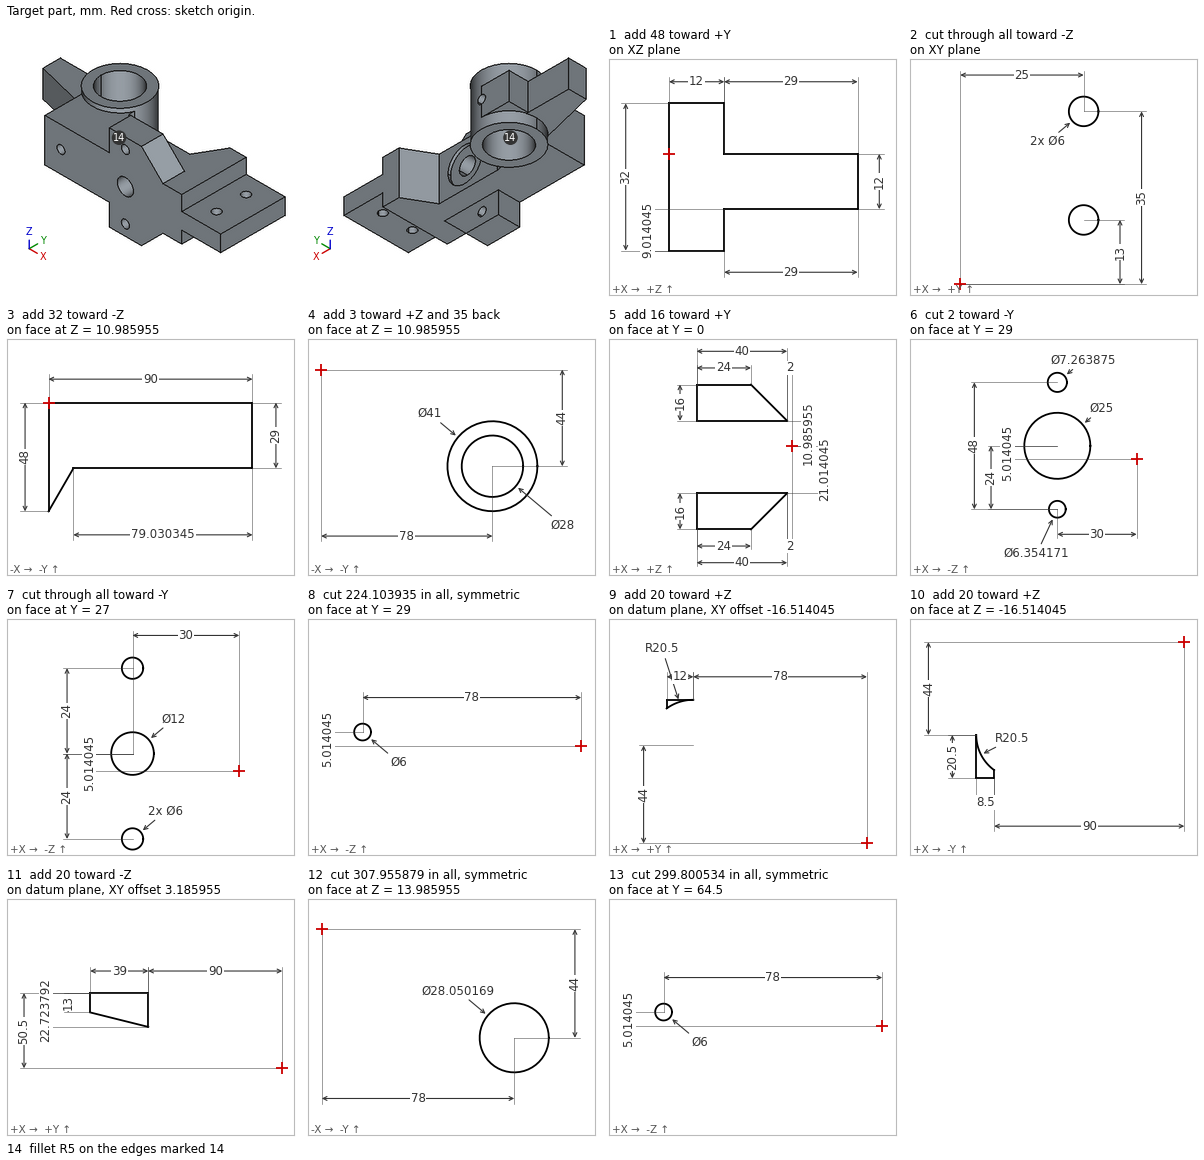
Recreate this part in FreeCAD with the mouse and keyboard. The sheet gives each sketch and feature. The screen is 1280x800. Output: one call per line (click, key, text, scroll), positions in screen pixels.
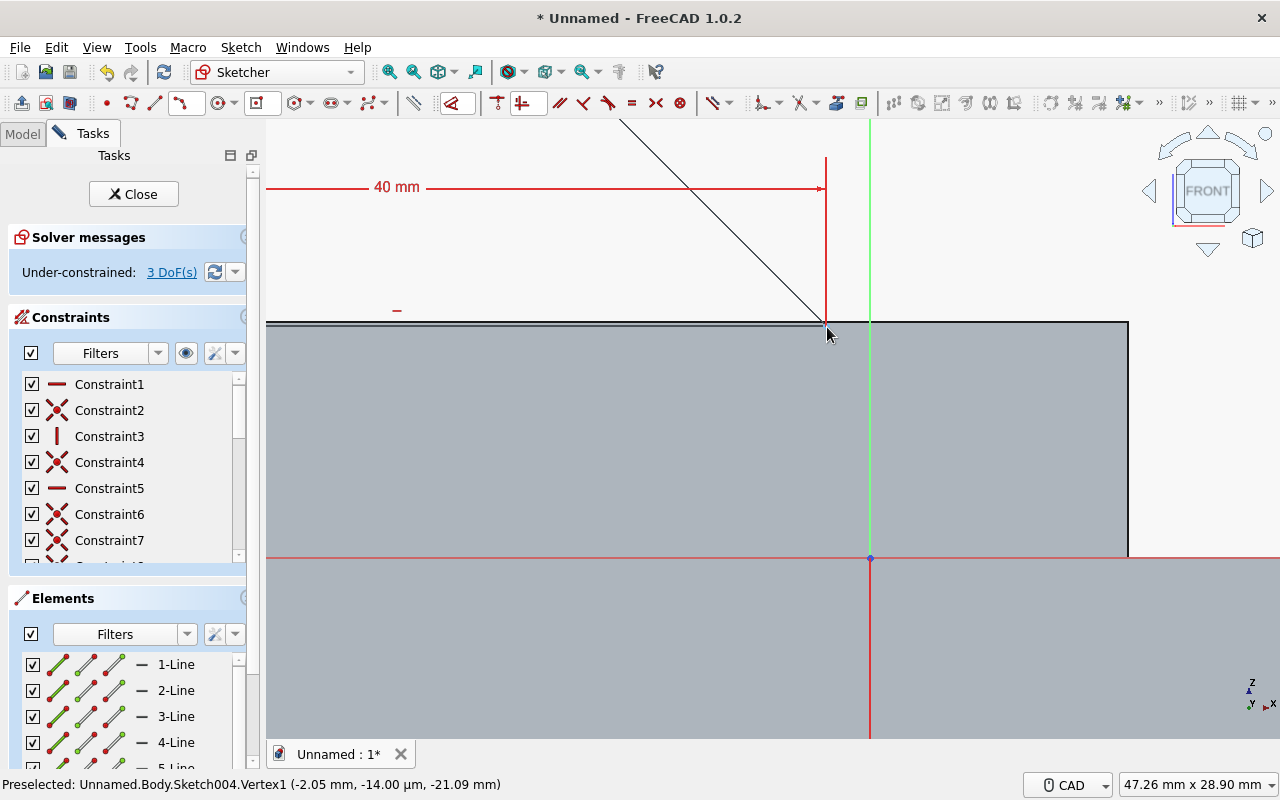
click(826, 326)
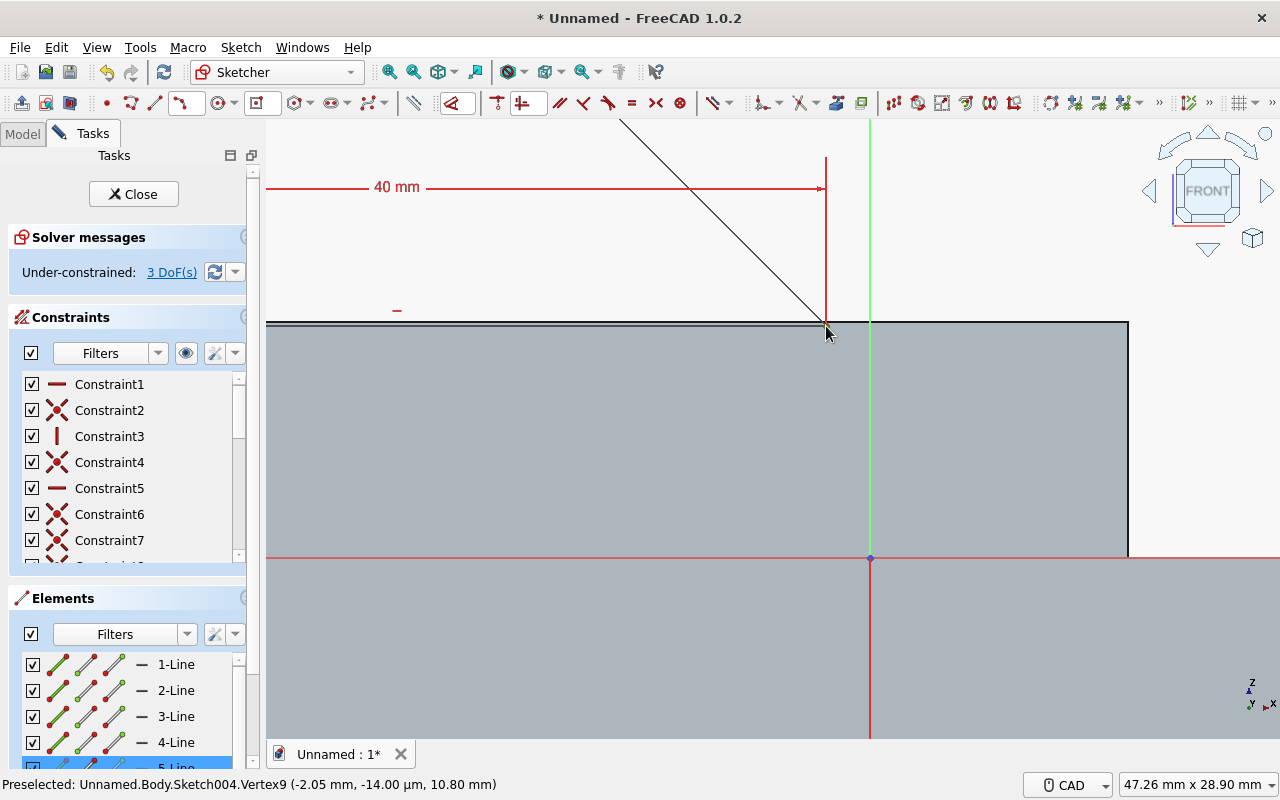
key(l)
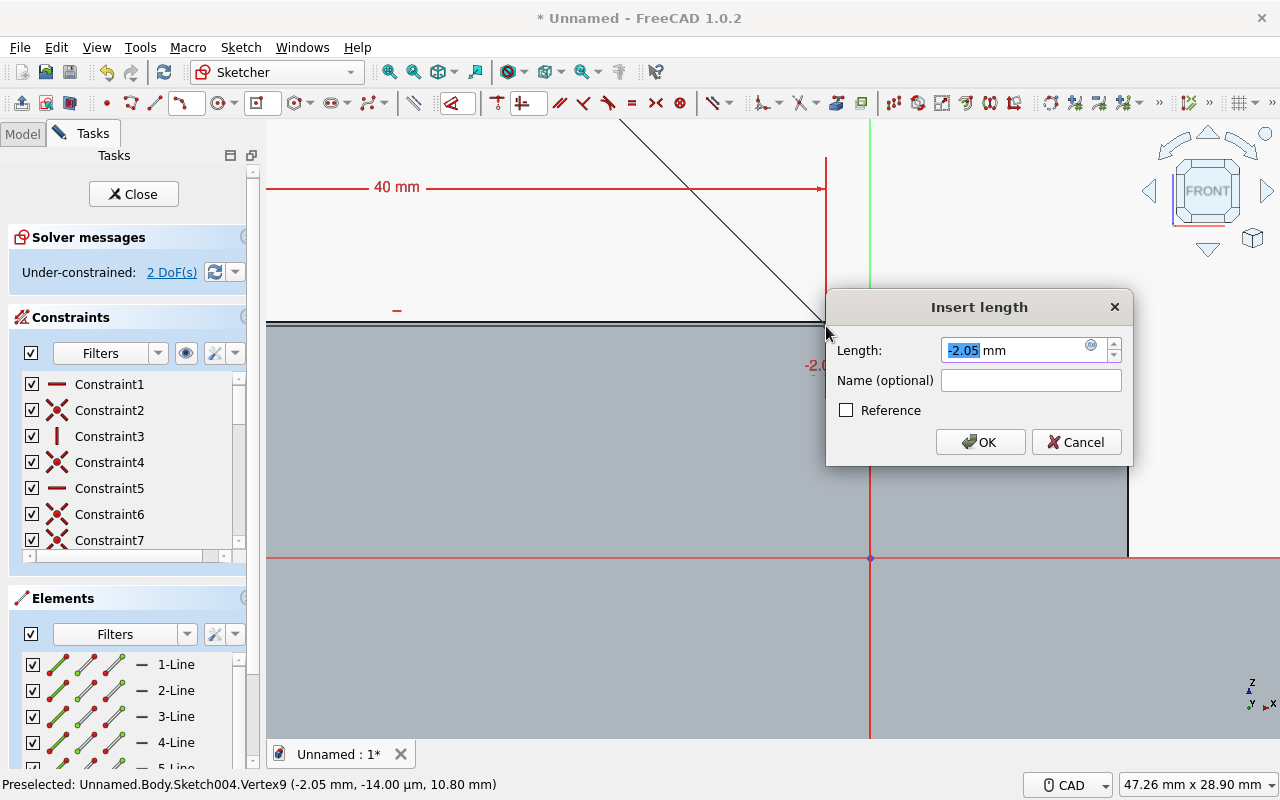
text(-2)
key(Return)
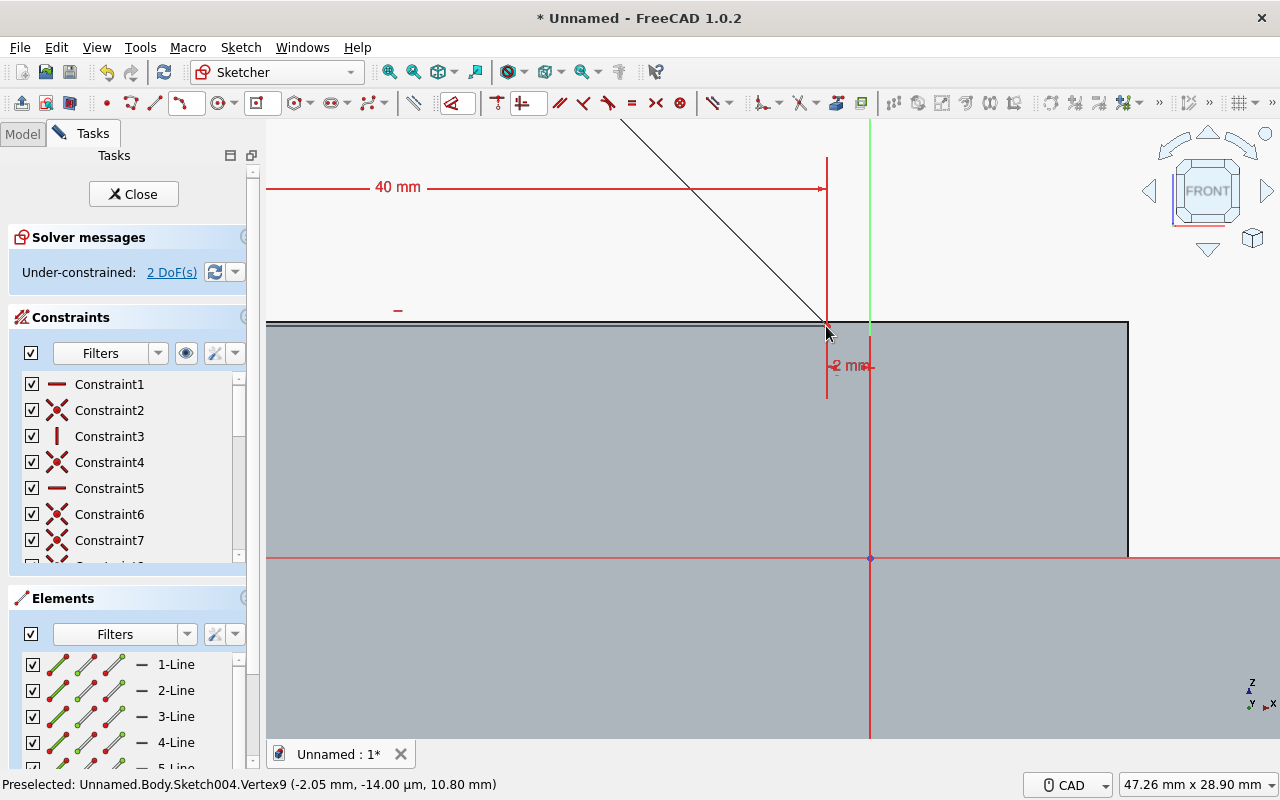
scroll(827, 327, down, 6)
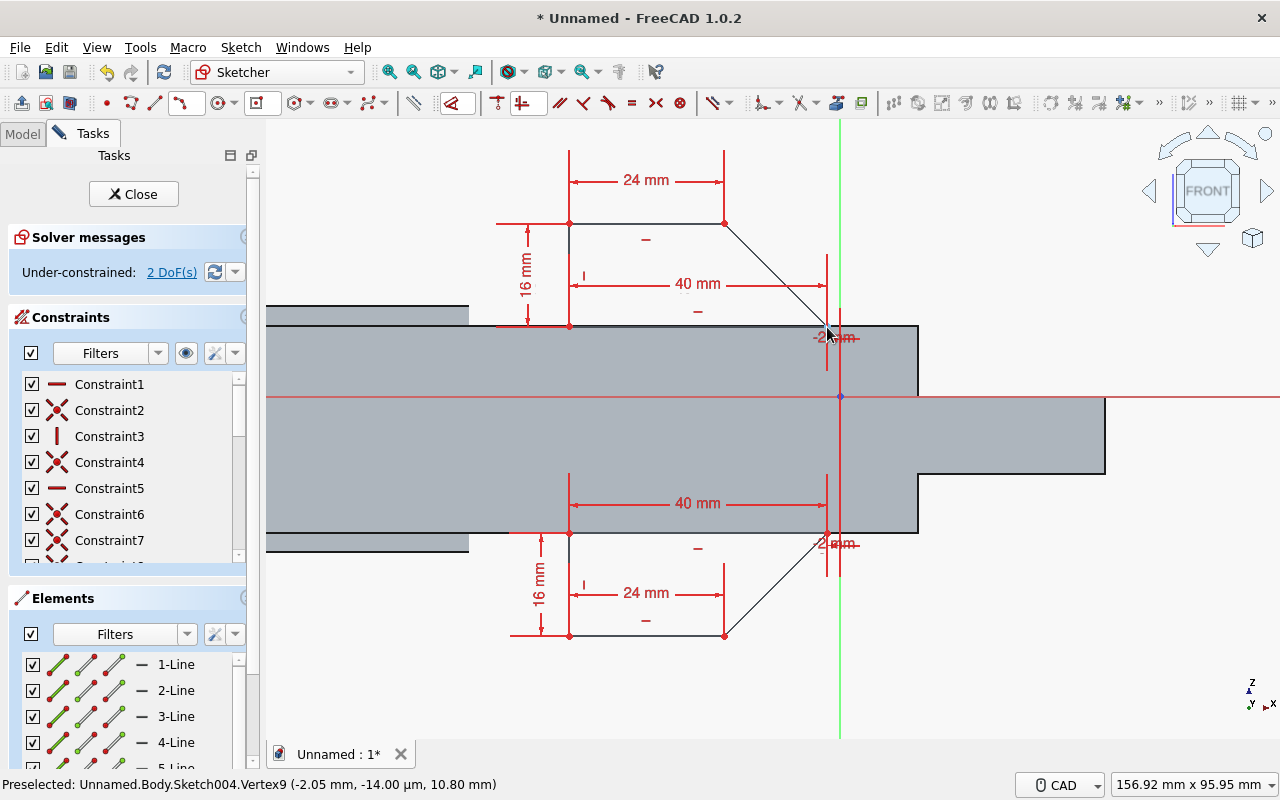
click(827, 533)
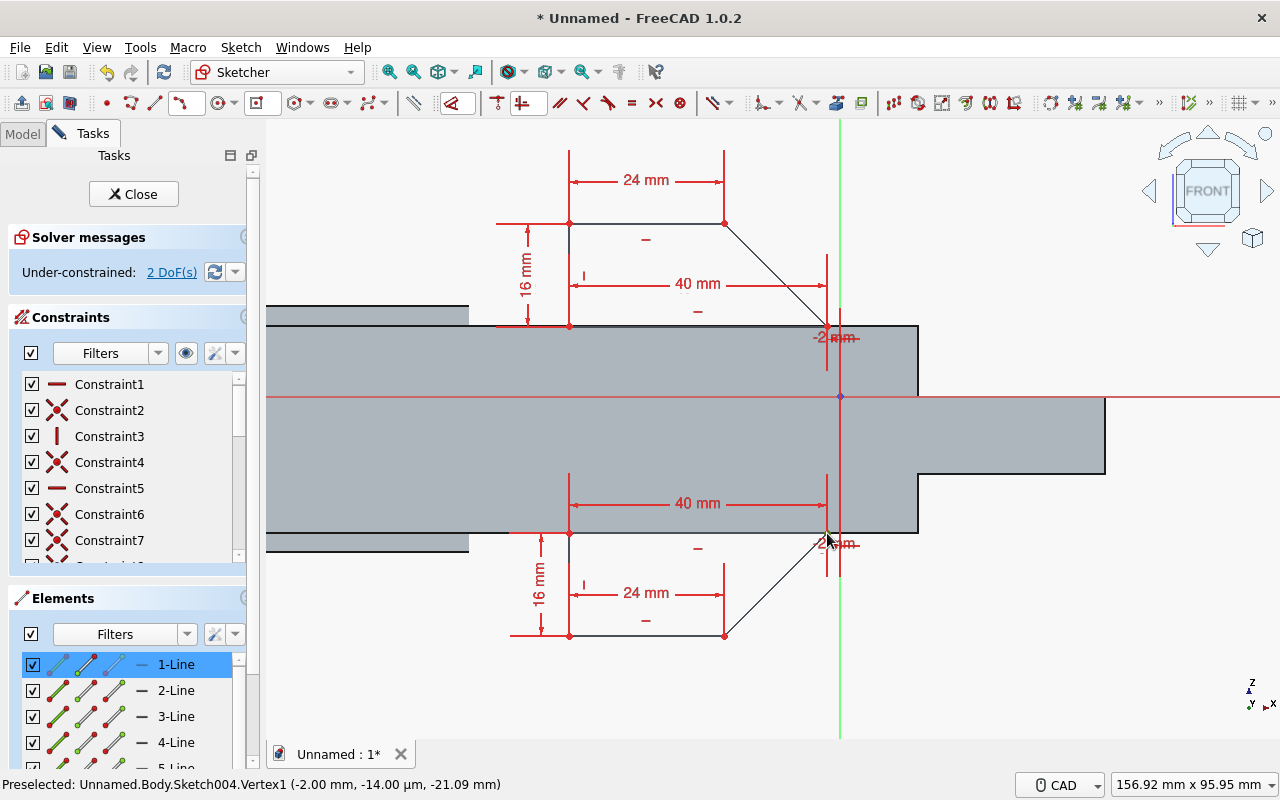
key(i)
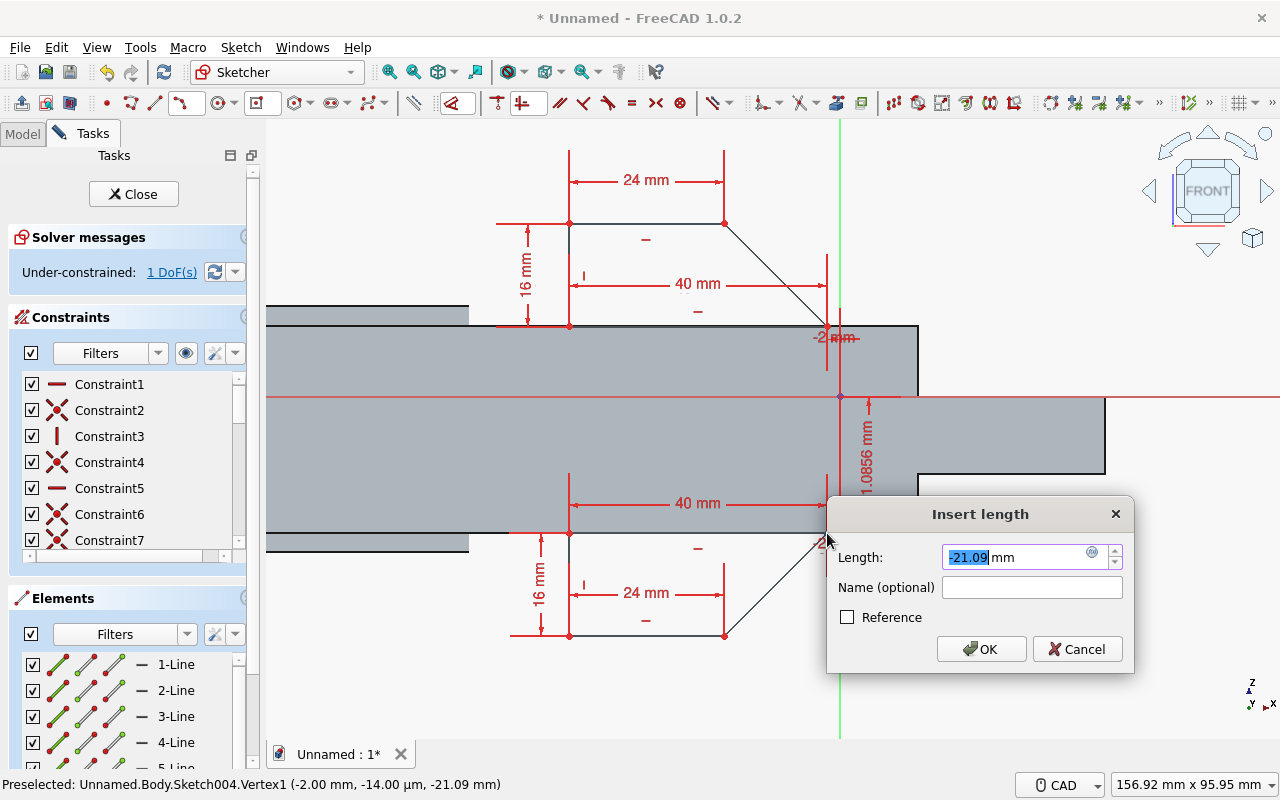
text(-21.014045)
key(Return)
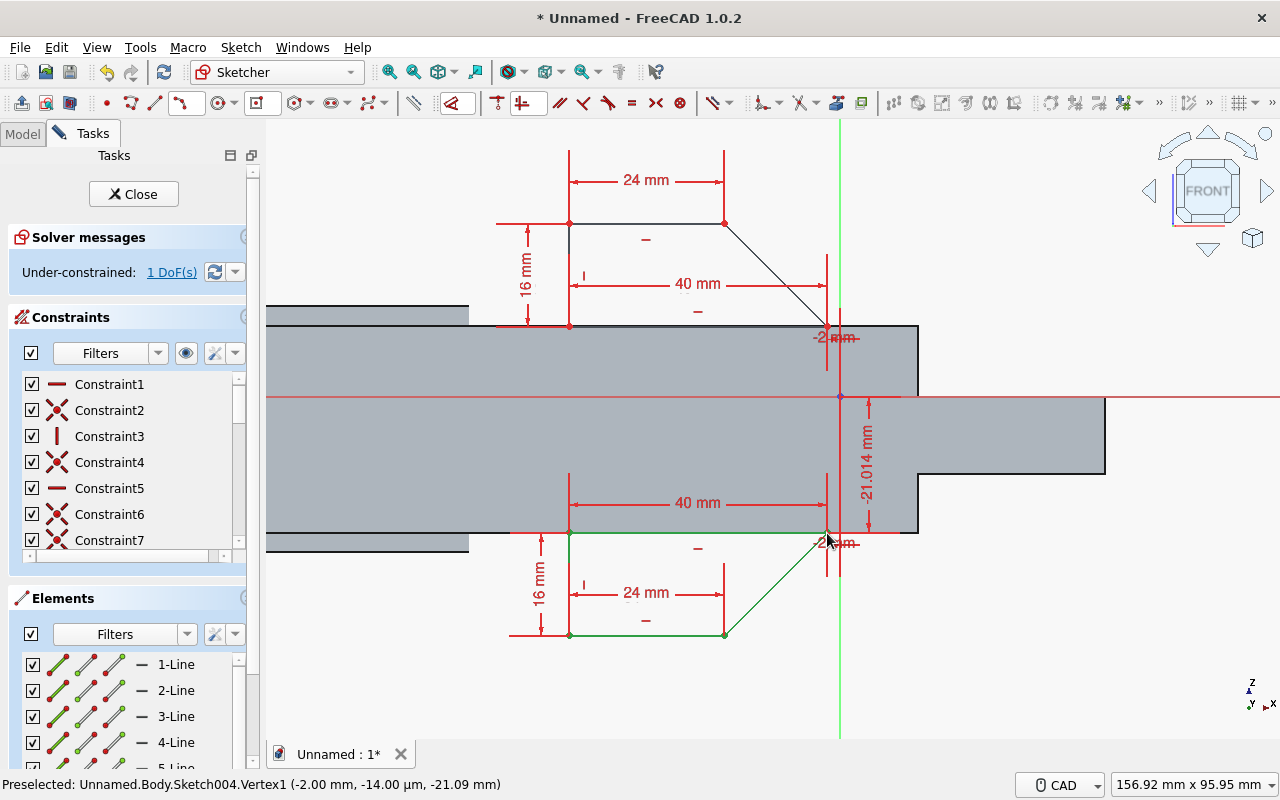
click(827, 327)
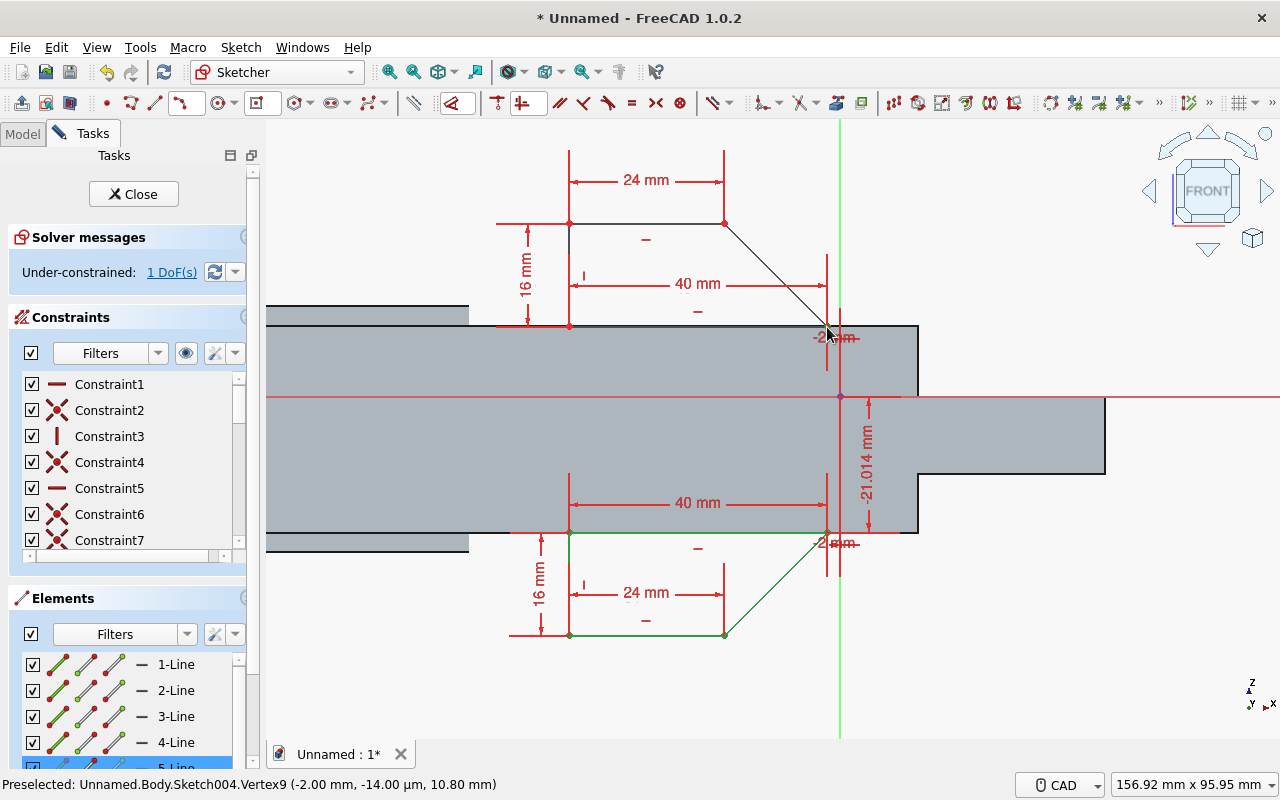
key(i)